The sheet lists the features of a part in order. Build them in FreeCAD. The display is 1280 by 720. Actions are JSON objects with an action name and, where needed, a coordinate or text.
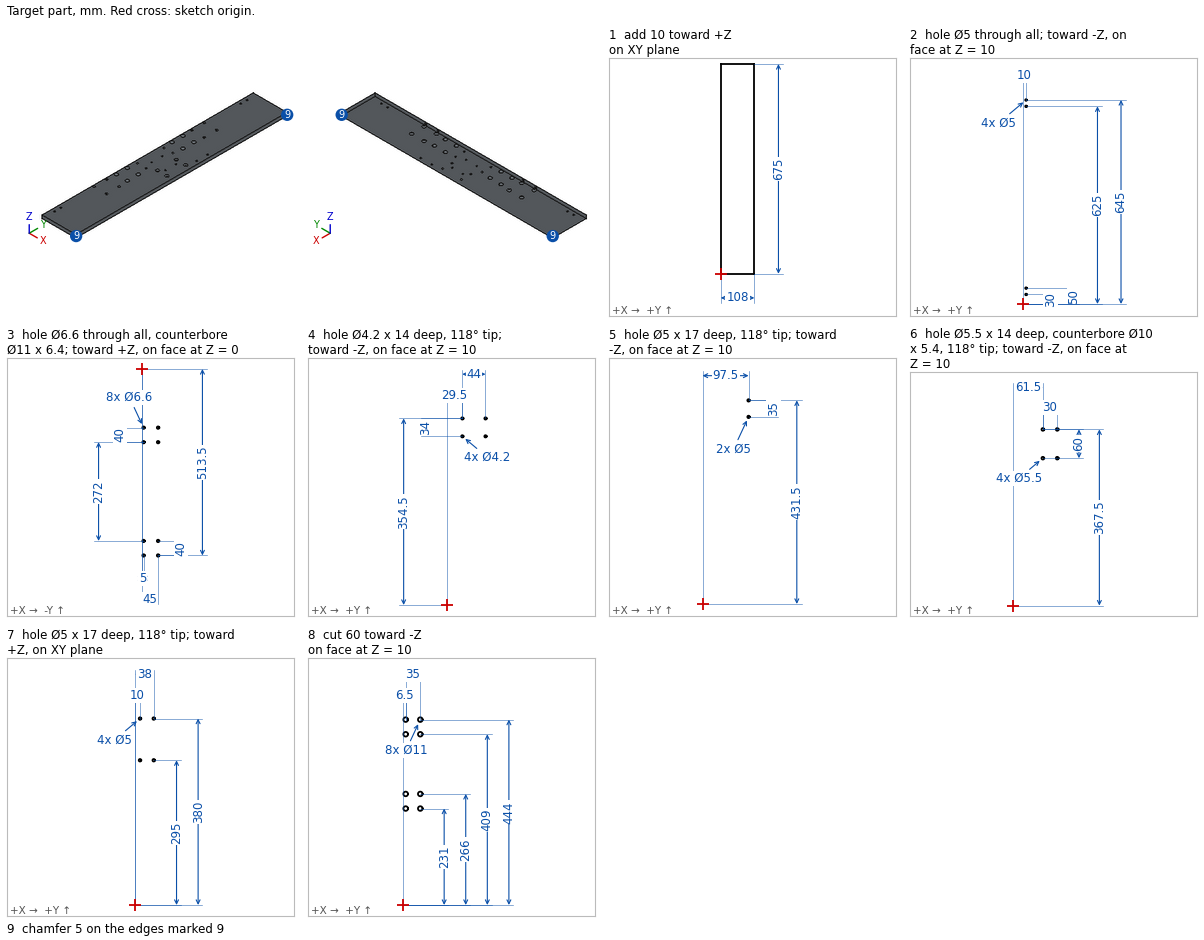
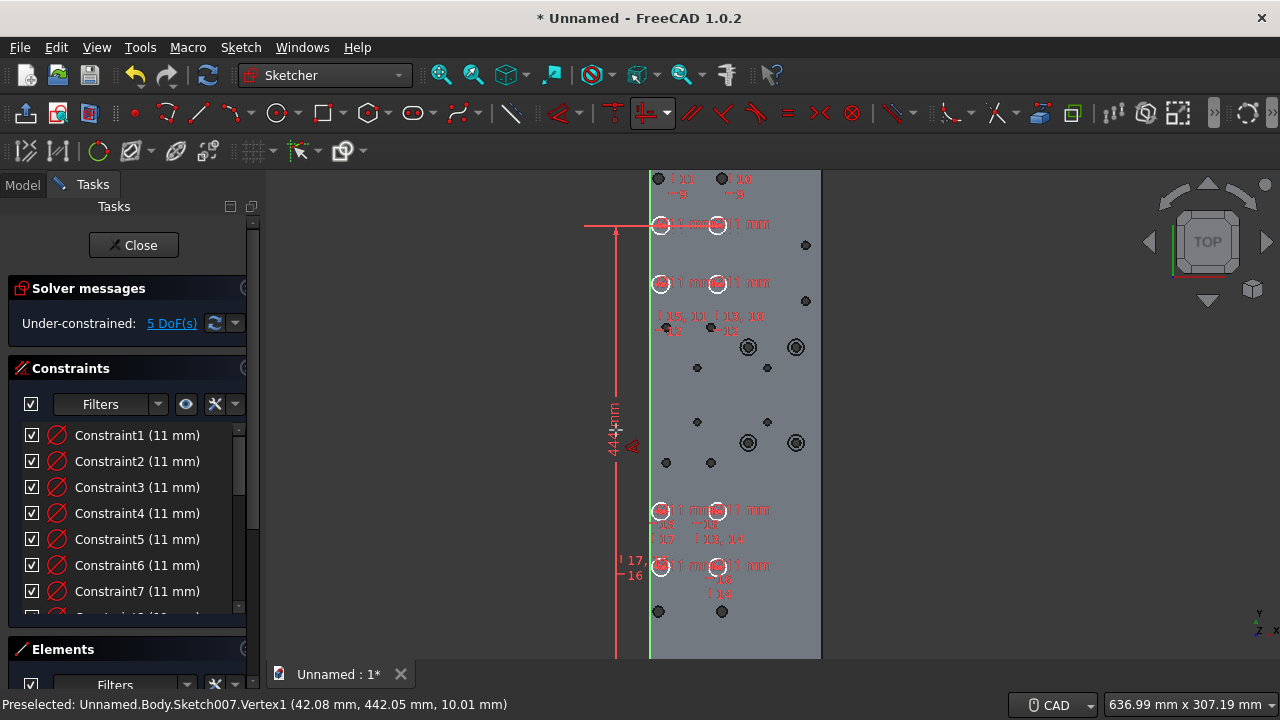
{"action": "scroll", "coordinate": [661, 226], "scroll_direction": "up", "scroll_amount": 7}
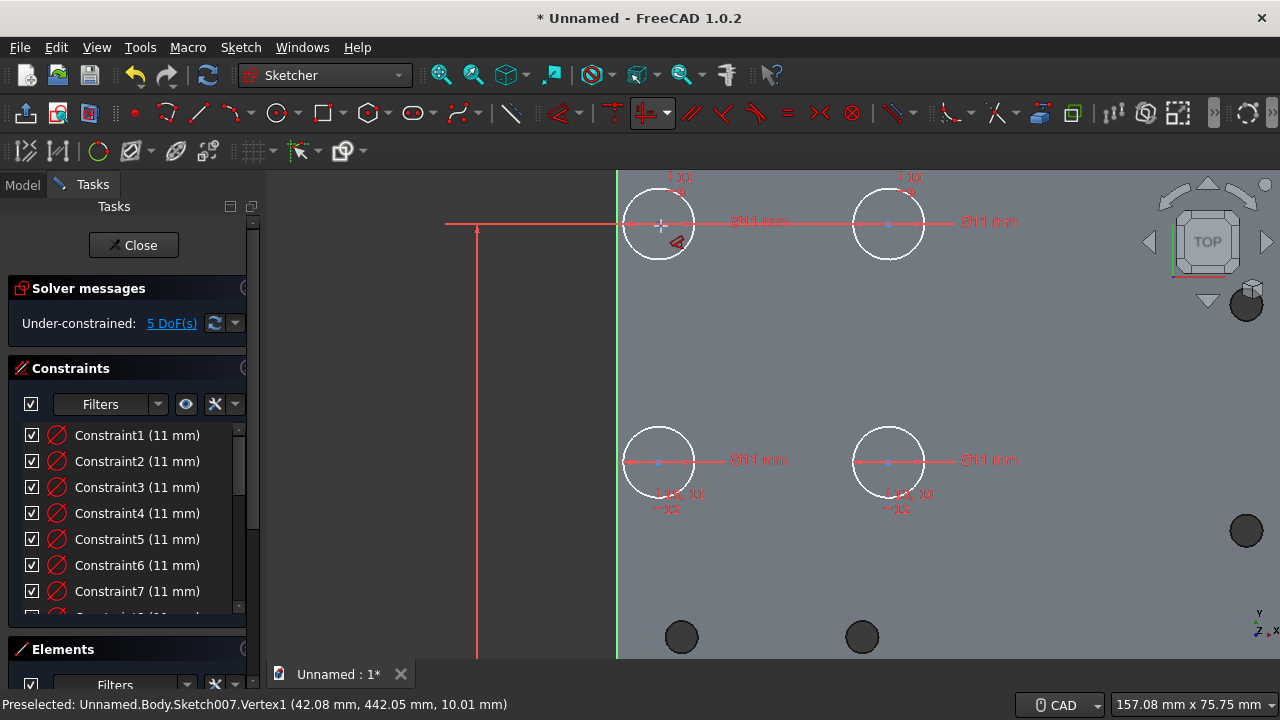
{"action": "left_click", "coordinate": [659, 224]}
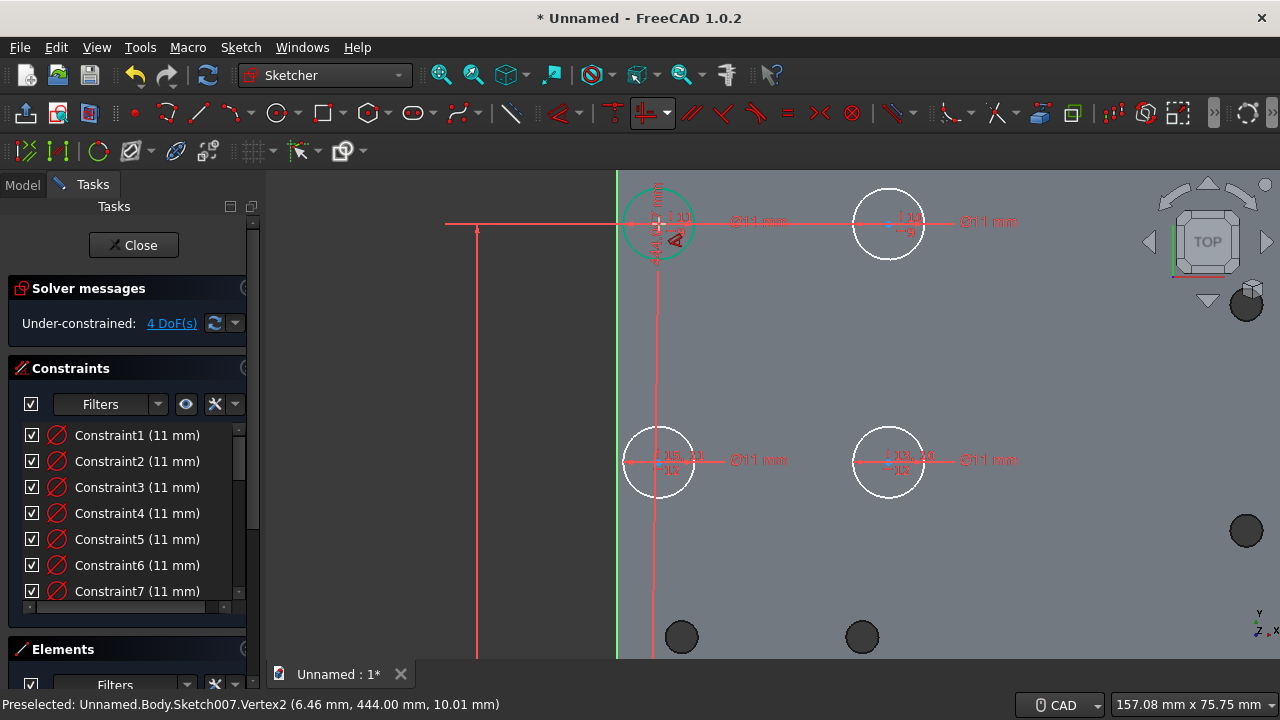
{"action": "key", "text": "Escape"}
{"action": "key", "text": "Escape"}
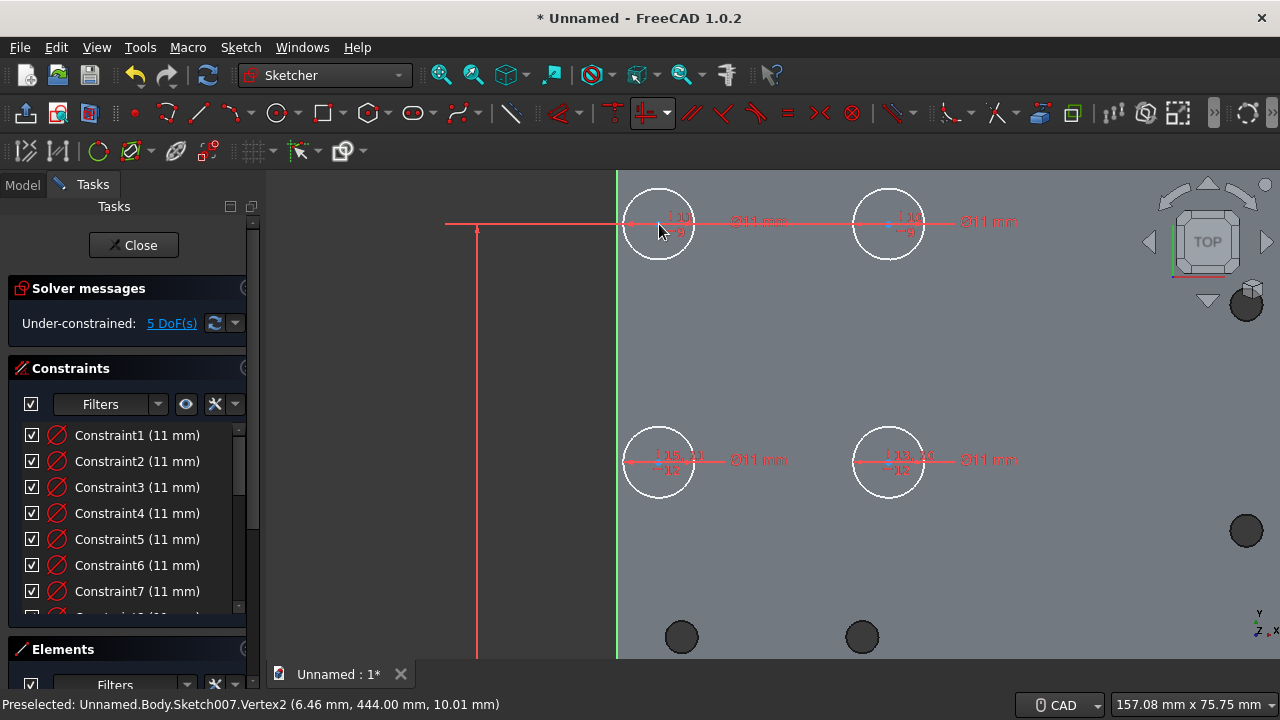
{"action": "left_click", "coordinate": [659, 224]}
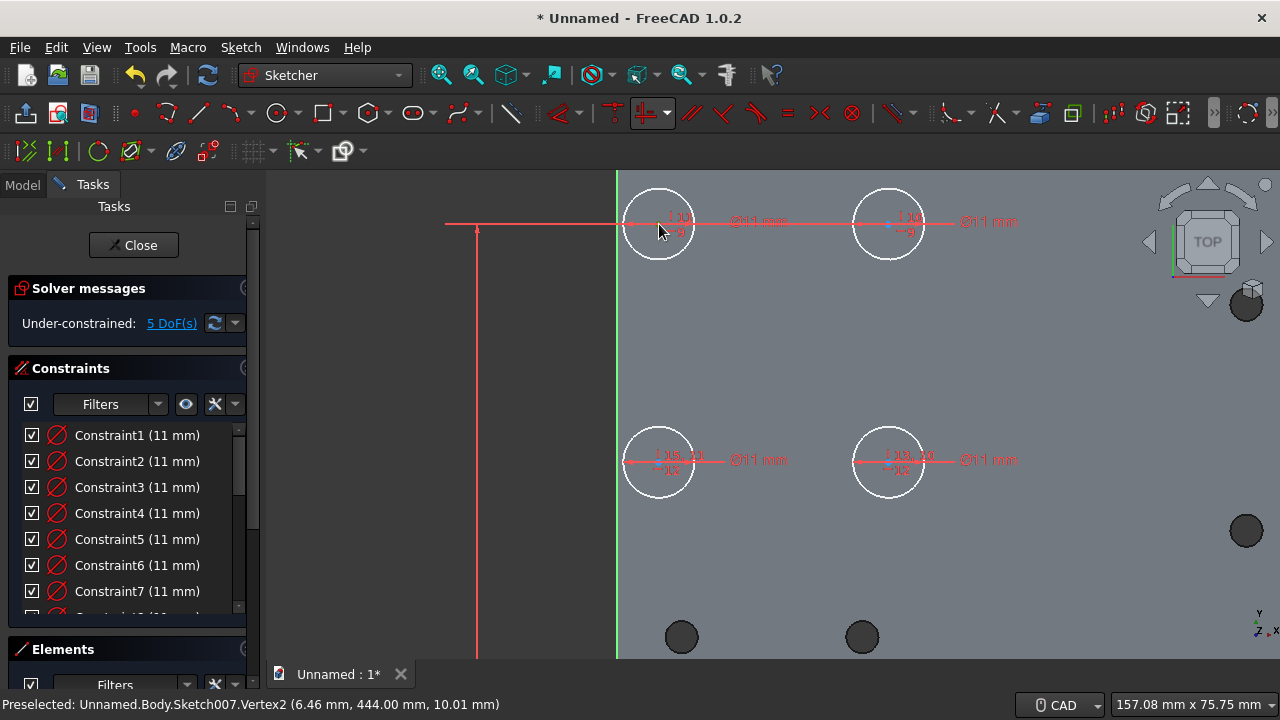
{"action": "left_click", "coordinate": [582, 114]}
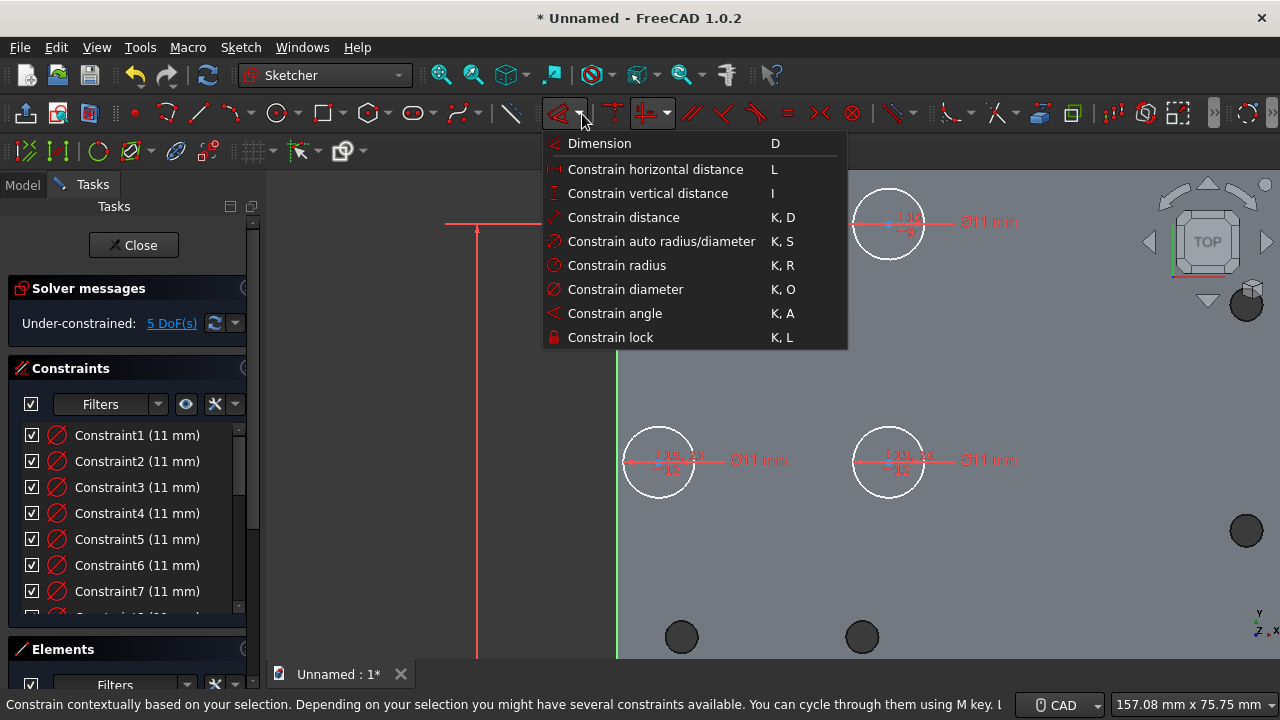
{"action": "left_click", "coordinate": [695, 169]}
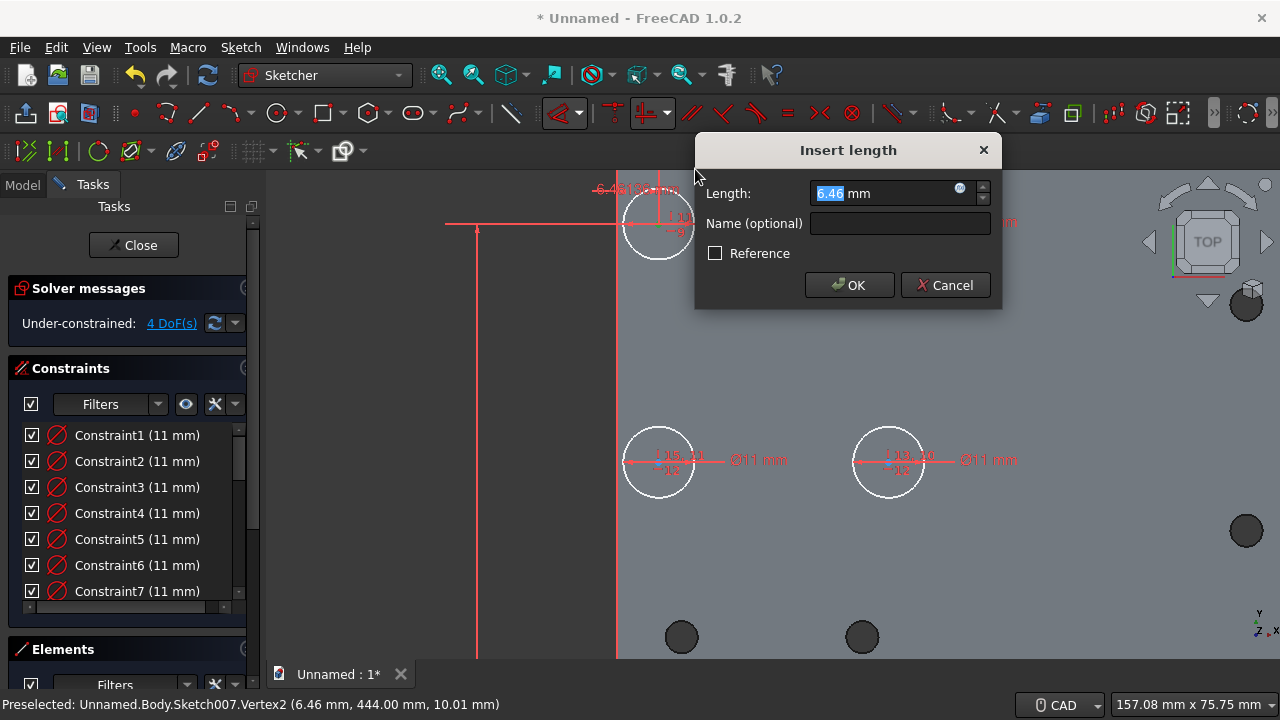
{"action": "type", "text": "6.5"}
{"action": "key", "text": "Return"}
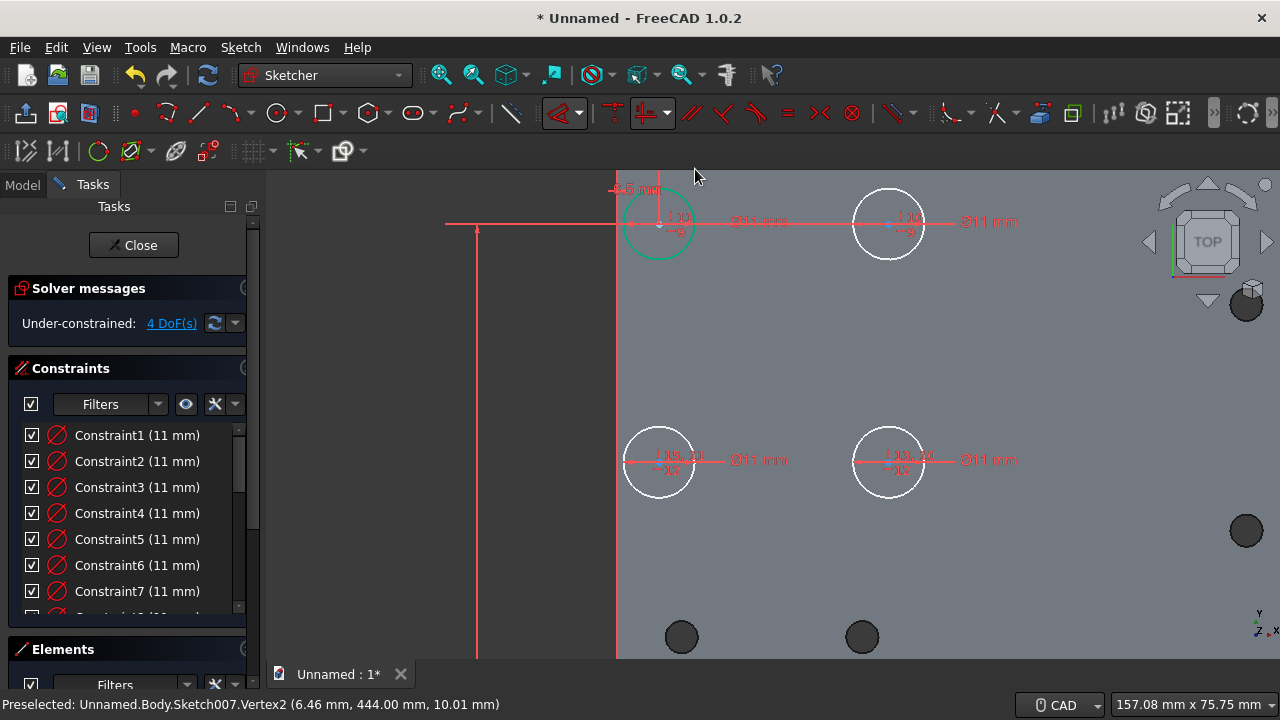
{"action": "scroll", "coordinate": [696, 262], "scroll_direction": "down", "scroll_amount": 11}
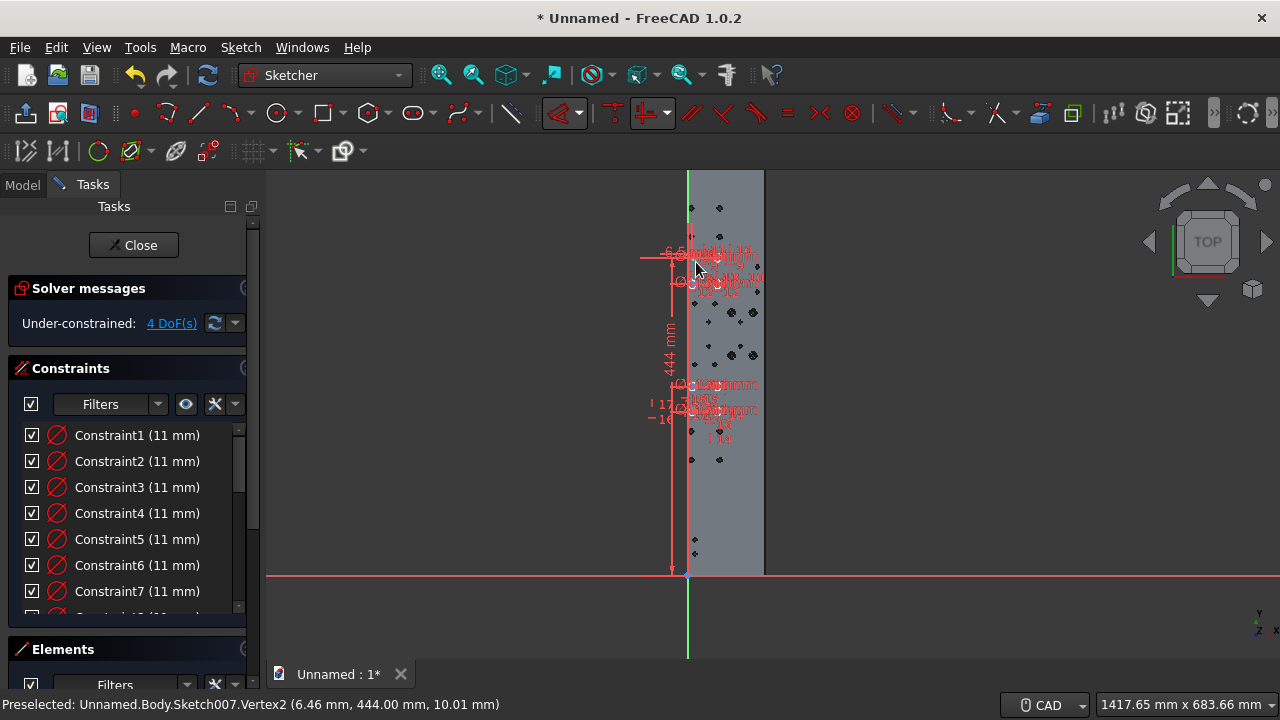
{"action": "left_click", "coordinate": [718, 284]}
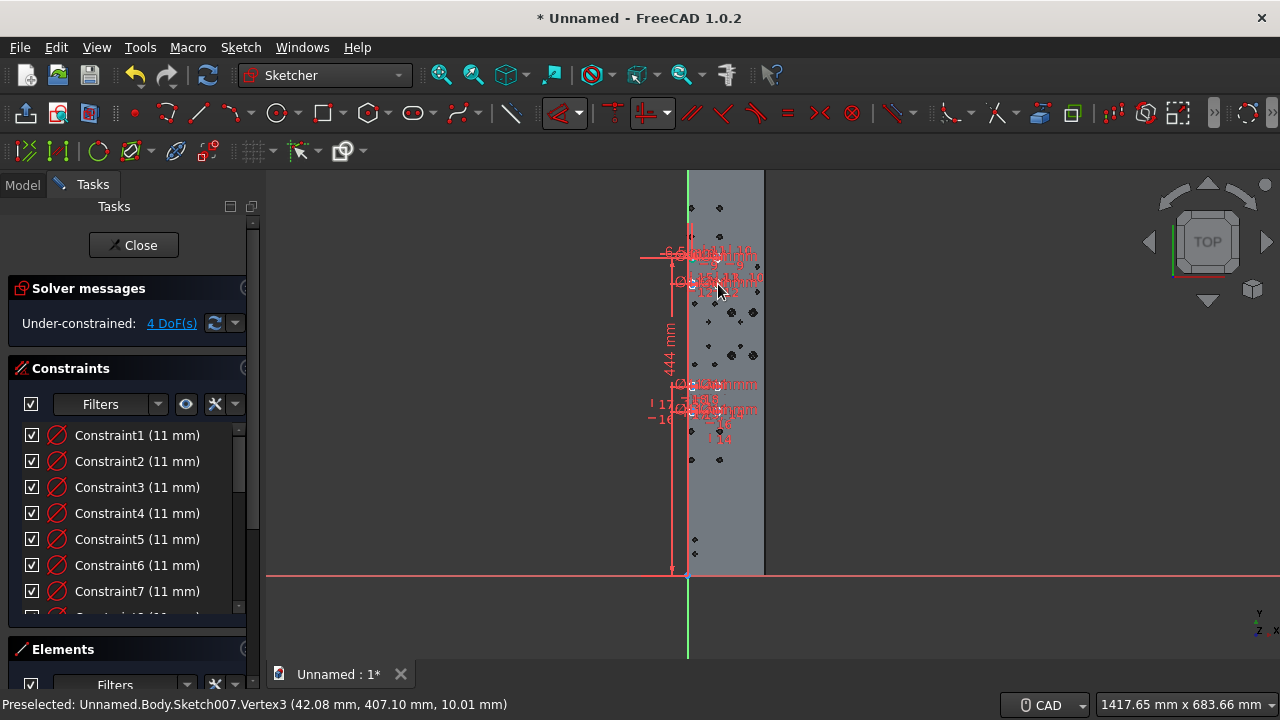
{"action": "left_click", "coordinate": [582, 114]}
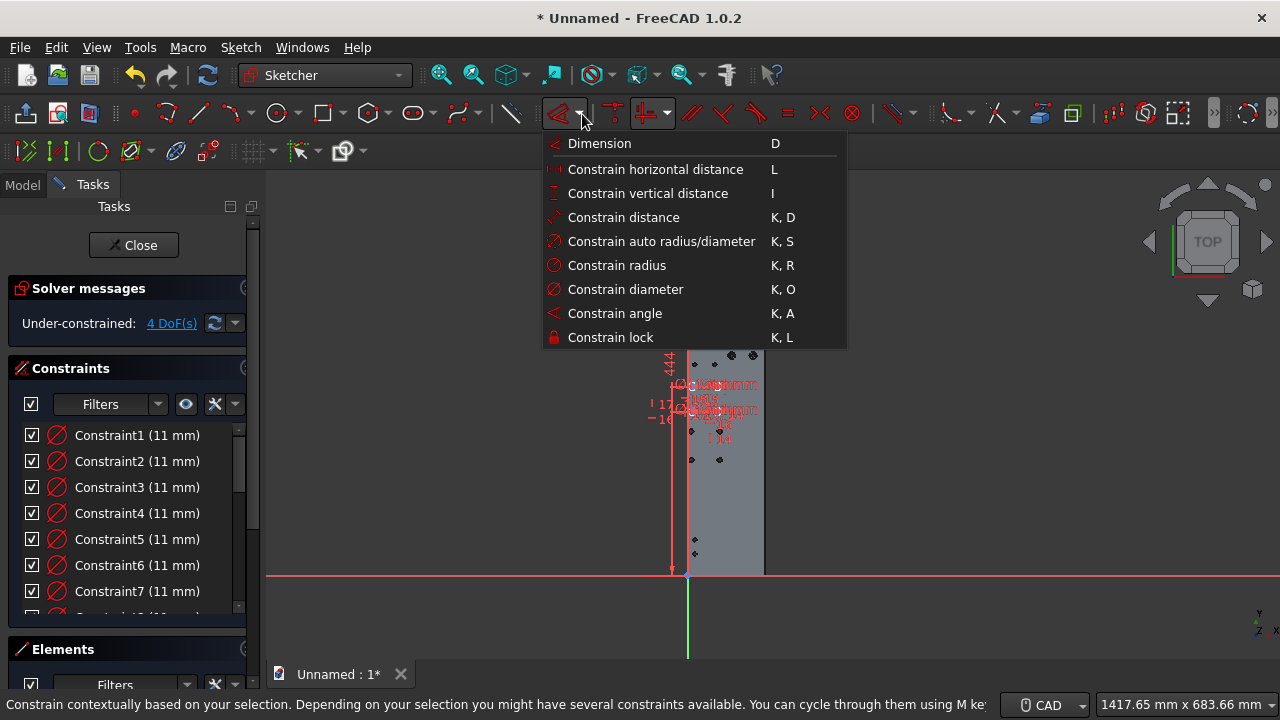
{"action": "left_click", "coordinate": [695, 193]}